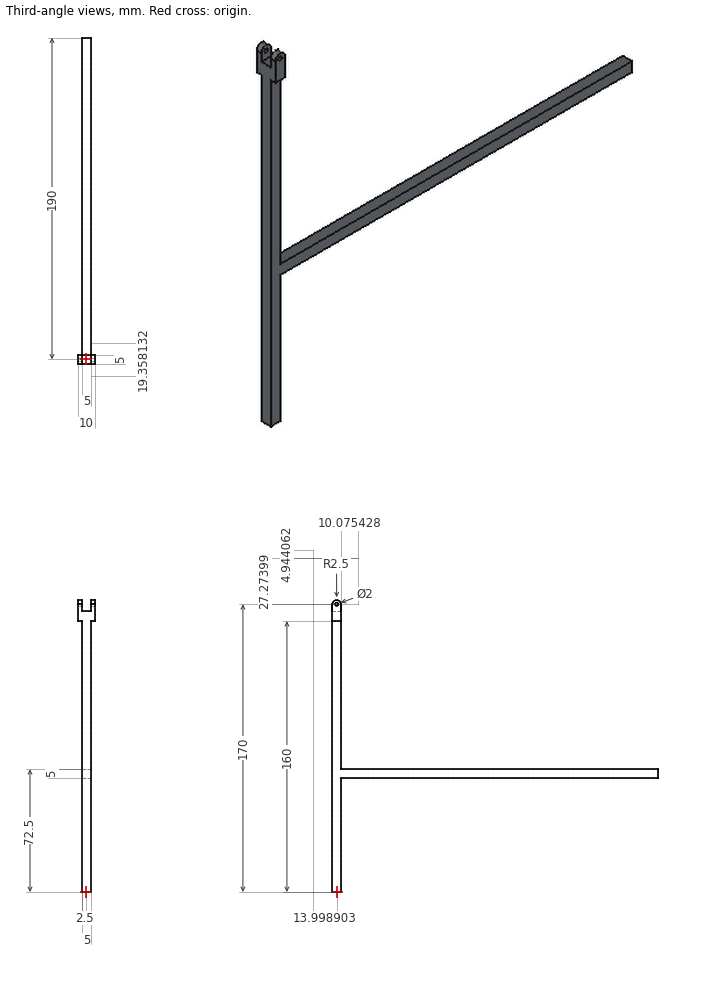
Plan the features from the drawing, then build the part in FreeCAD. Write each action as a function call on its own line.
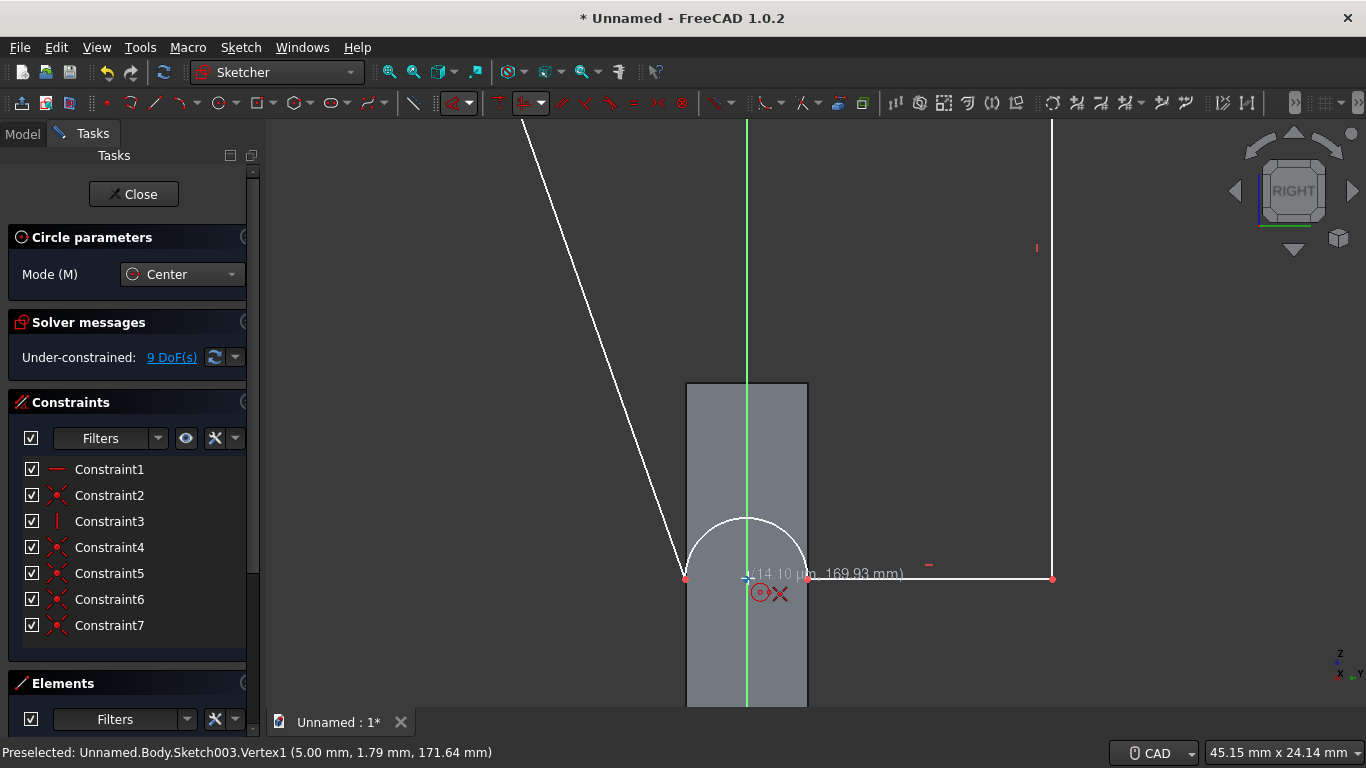
click(747, 578)
click(764, 560)
key(Escape)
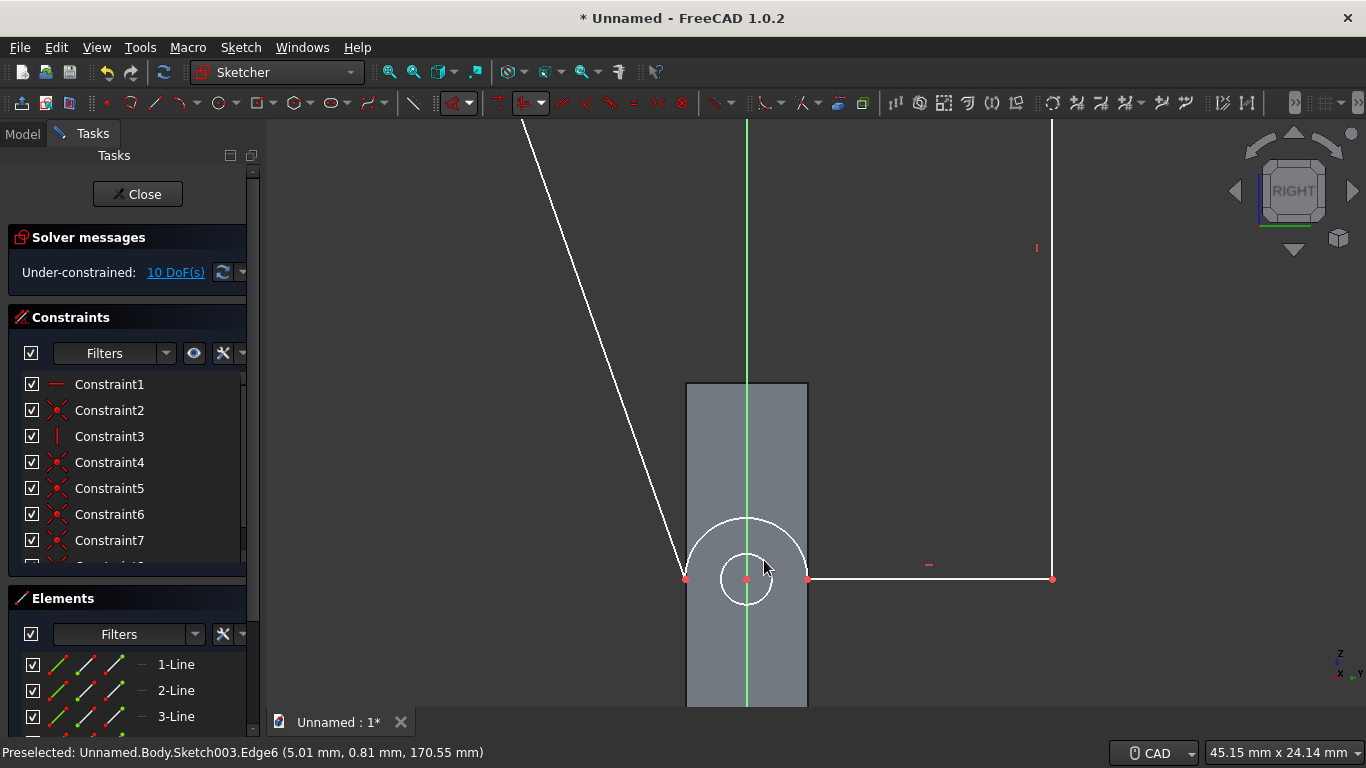
click(746, 579)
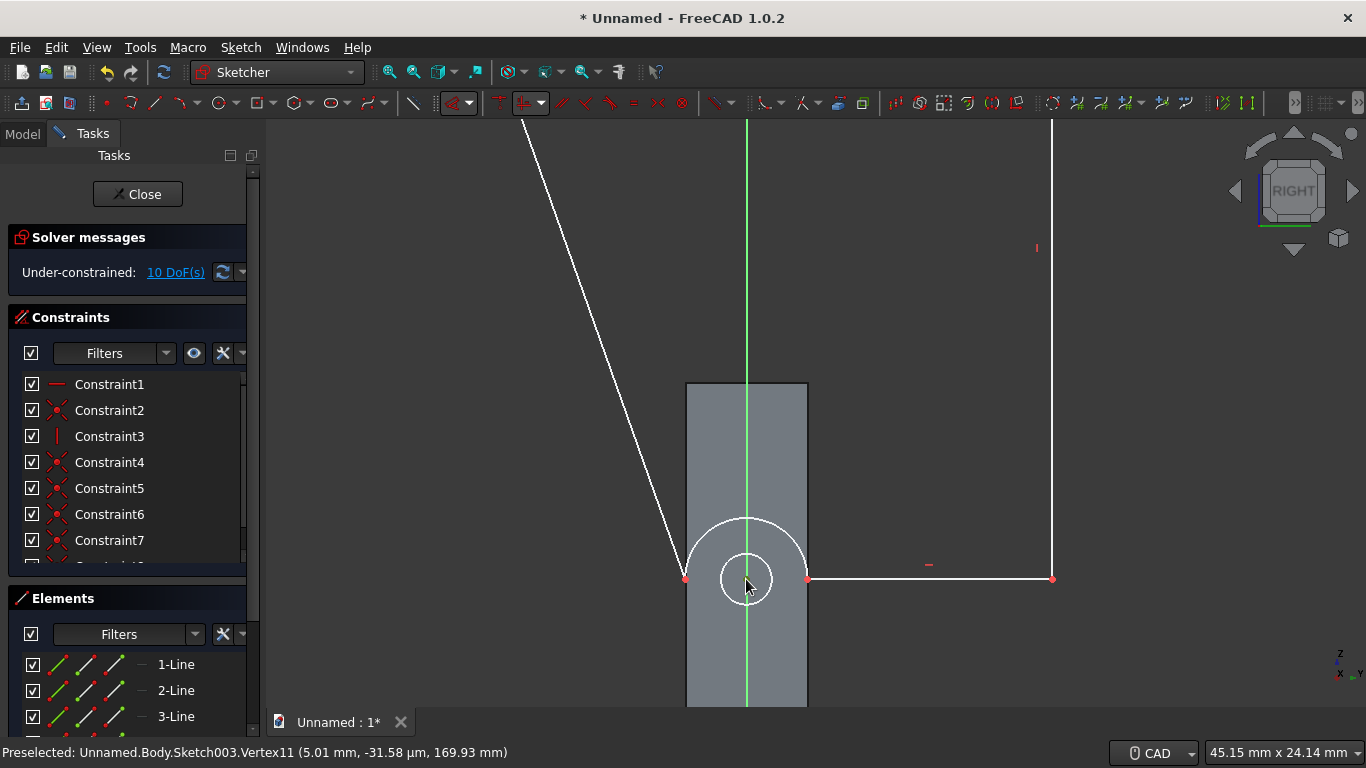
click(747, 641)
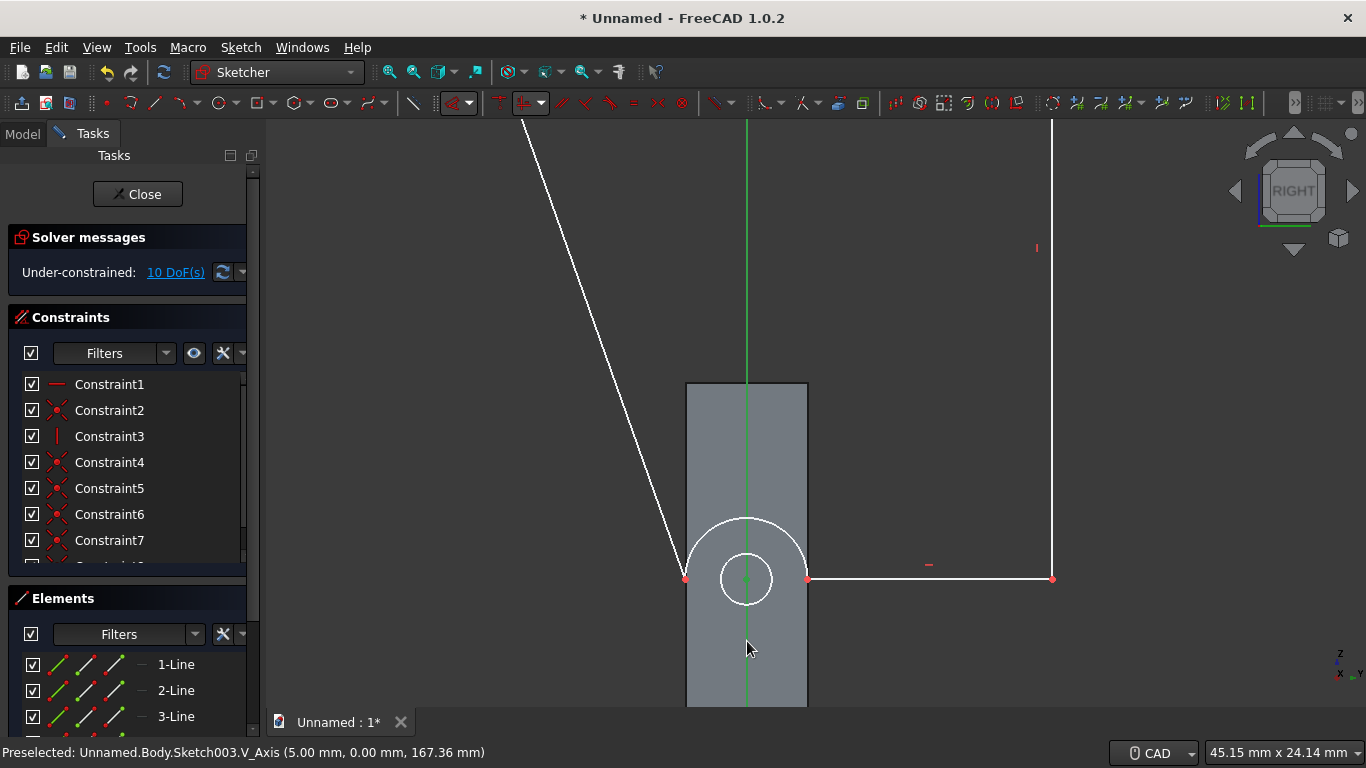
click(500, 104)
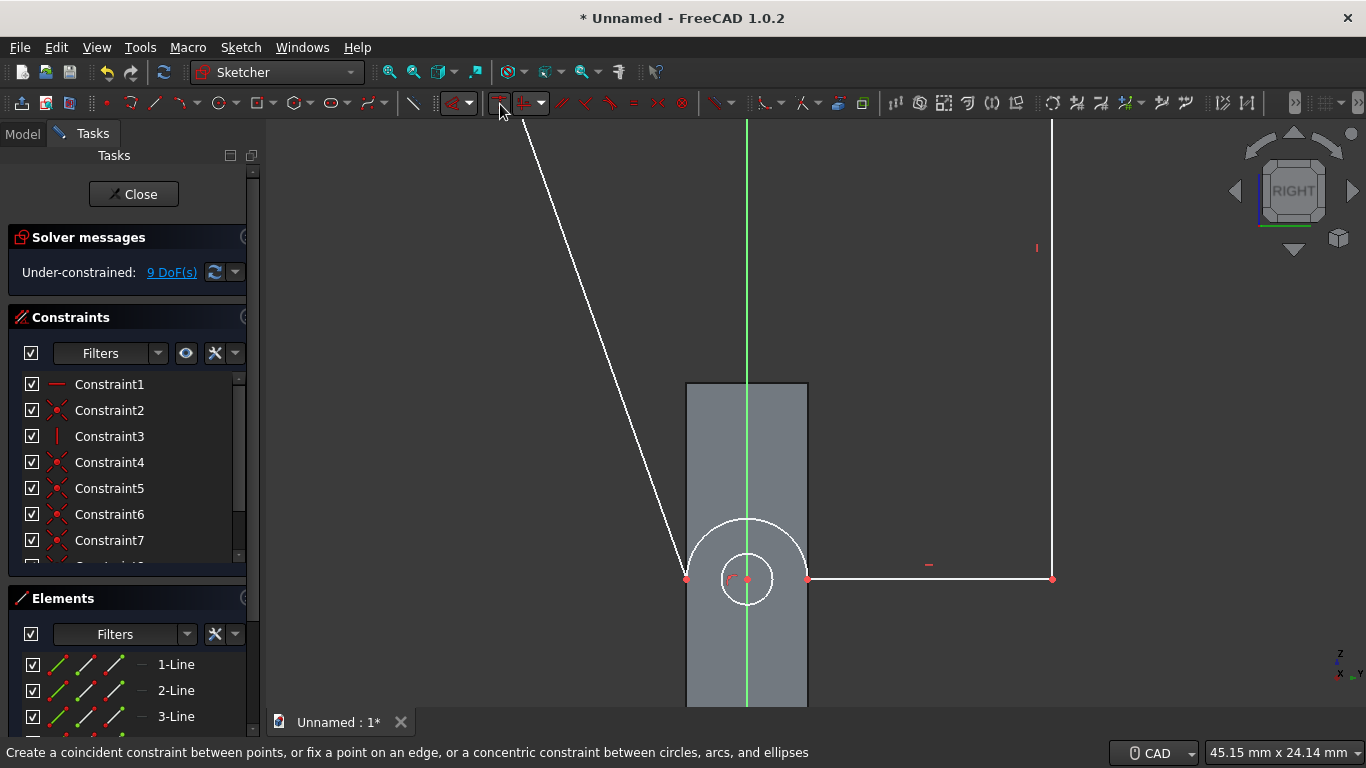
click(783, 530)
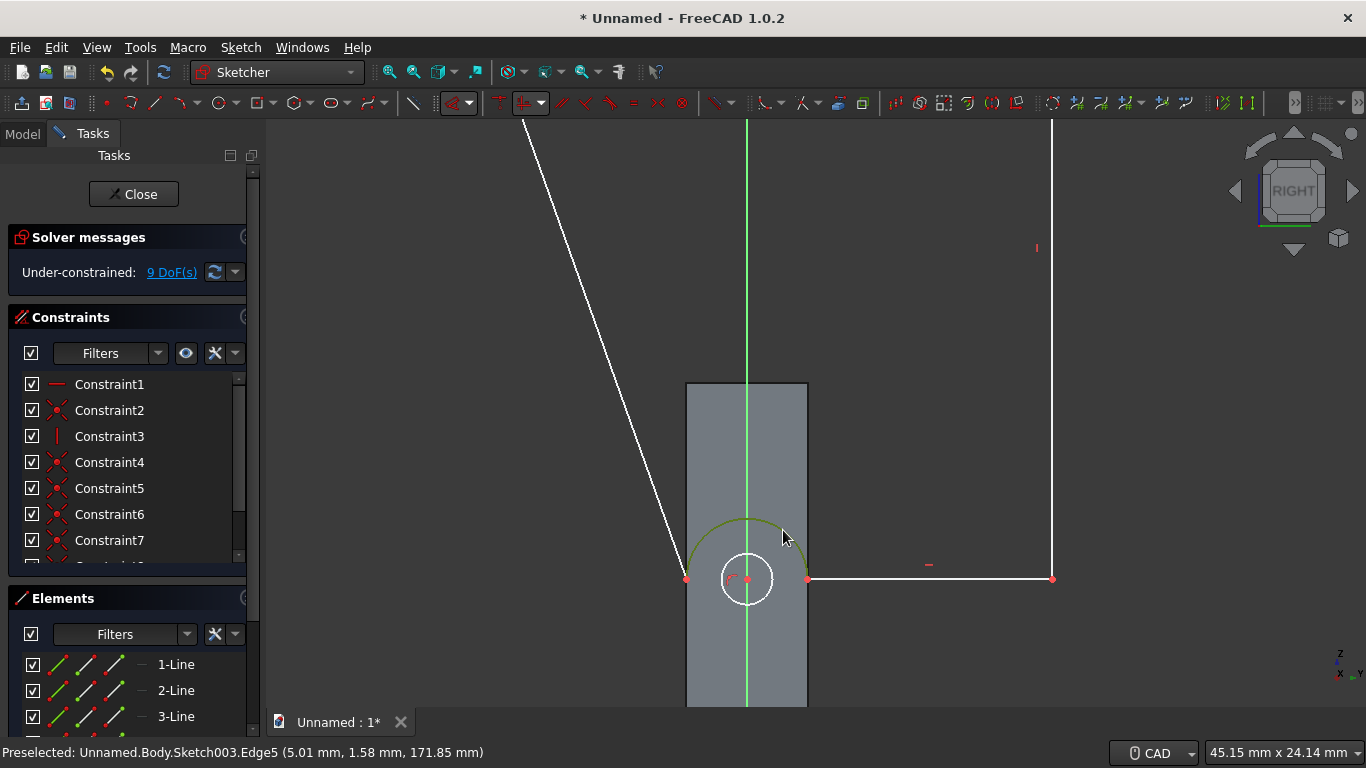
click(472, 104)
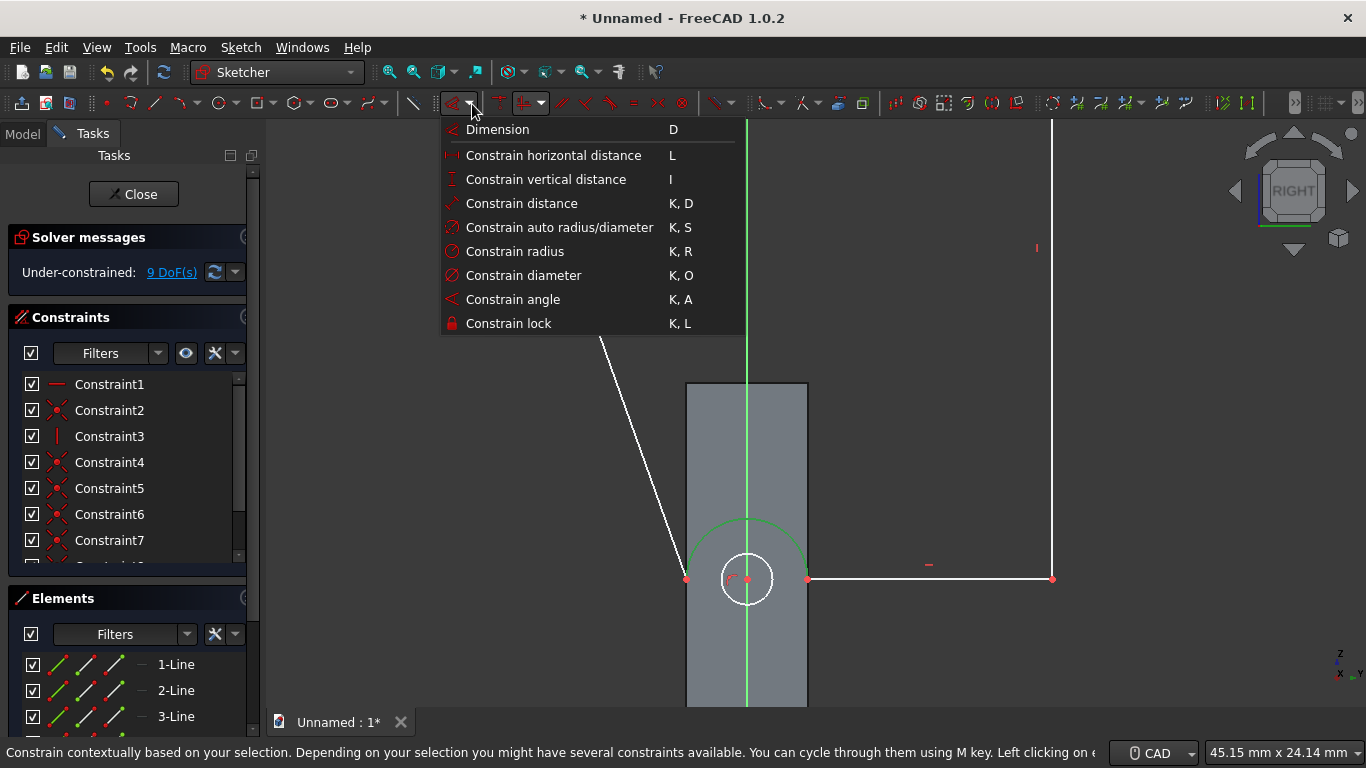
click(593, 251)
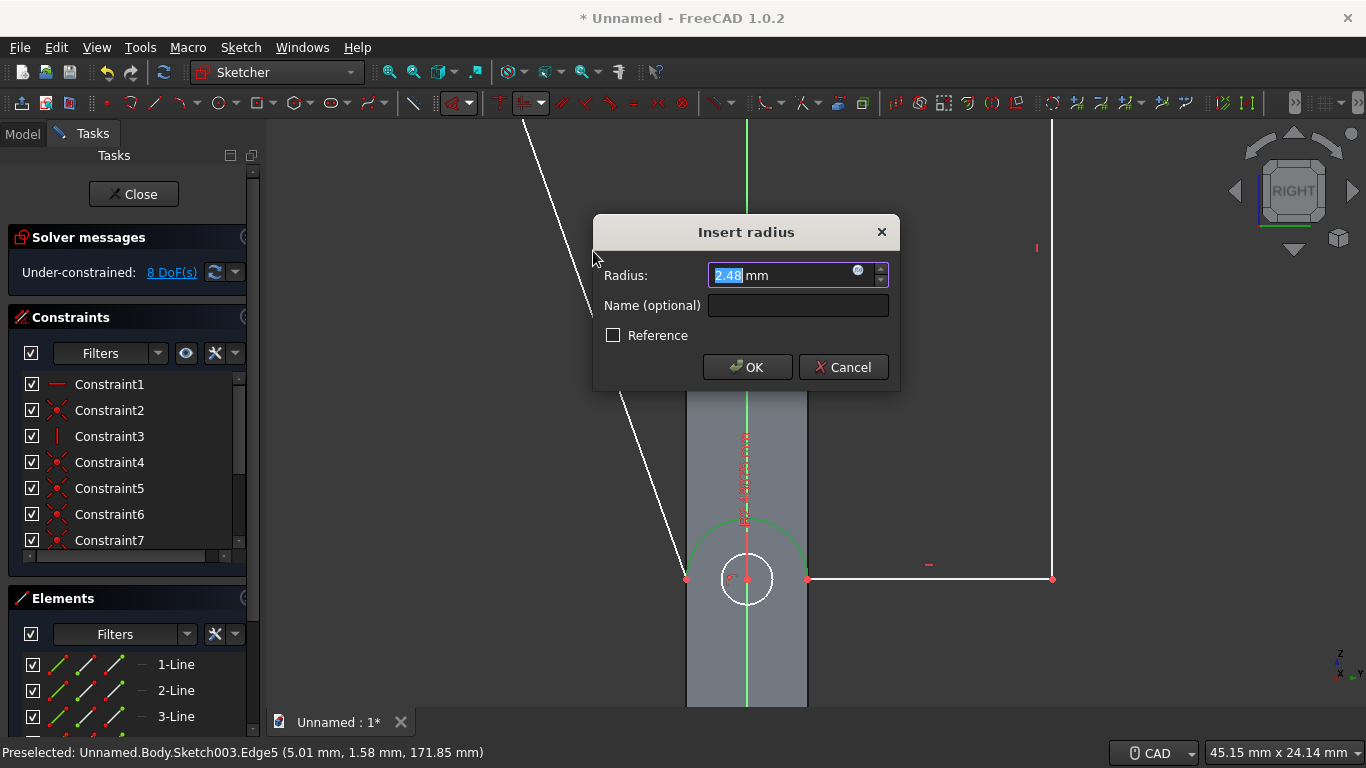
text(2.5)
key(Return)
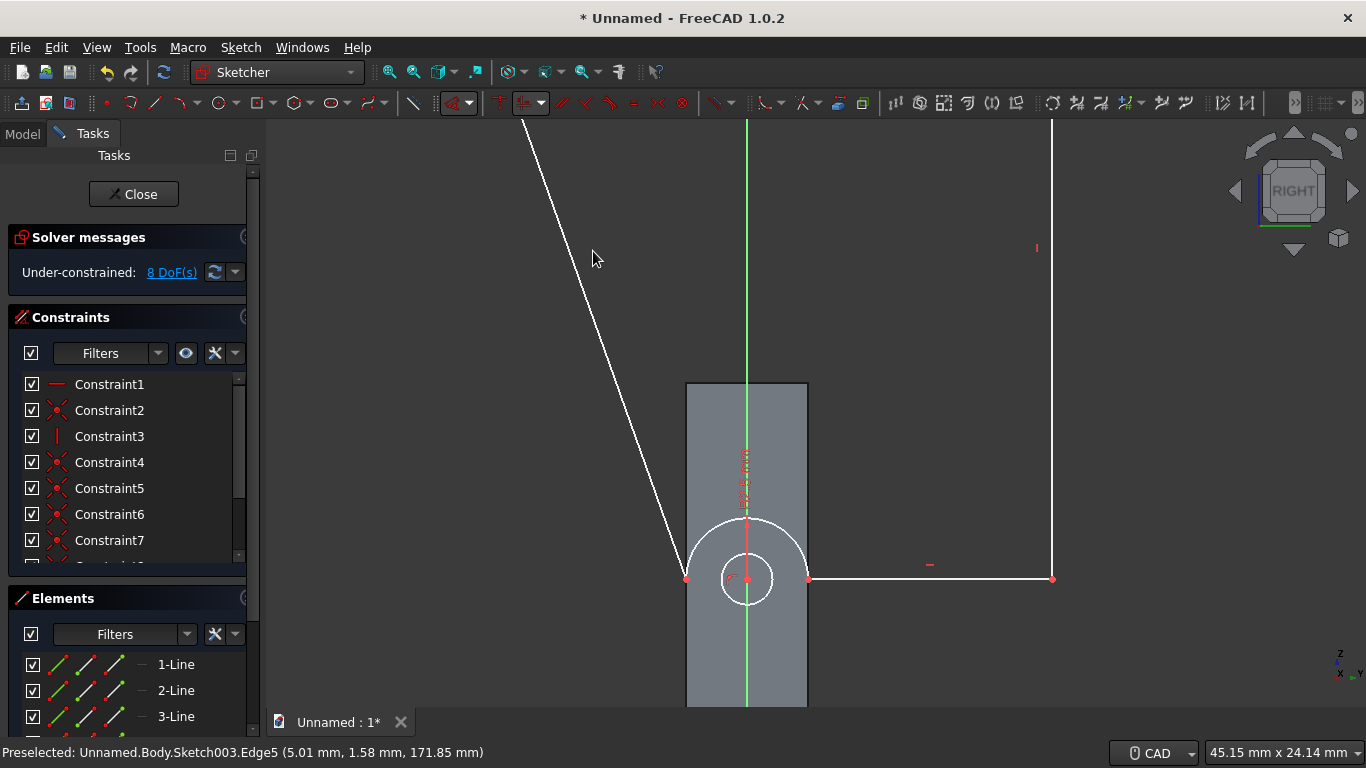
click(765, 561)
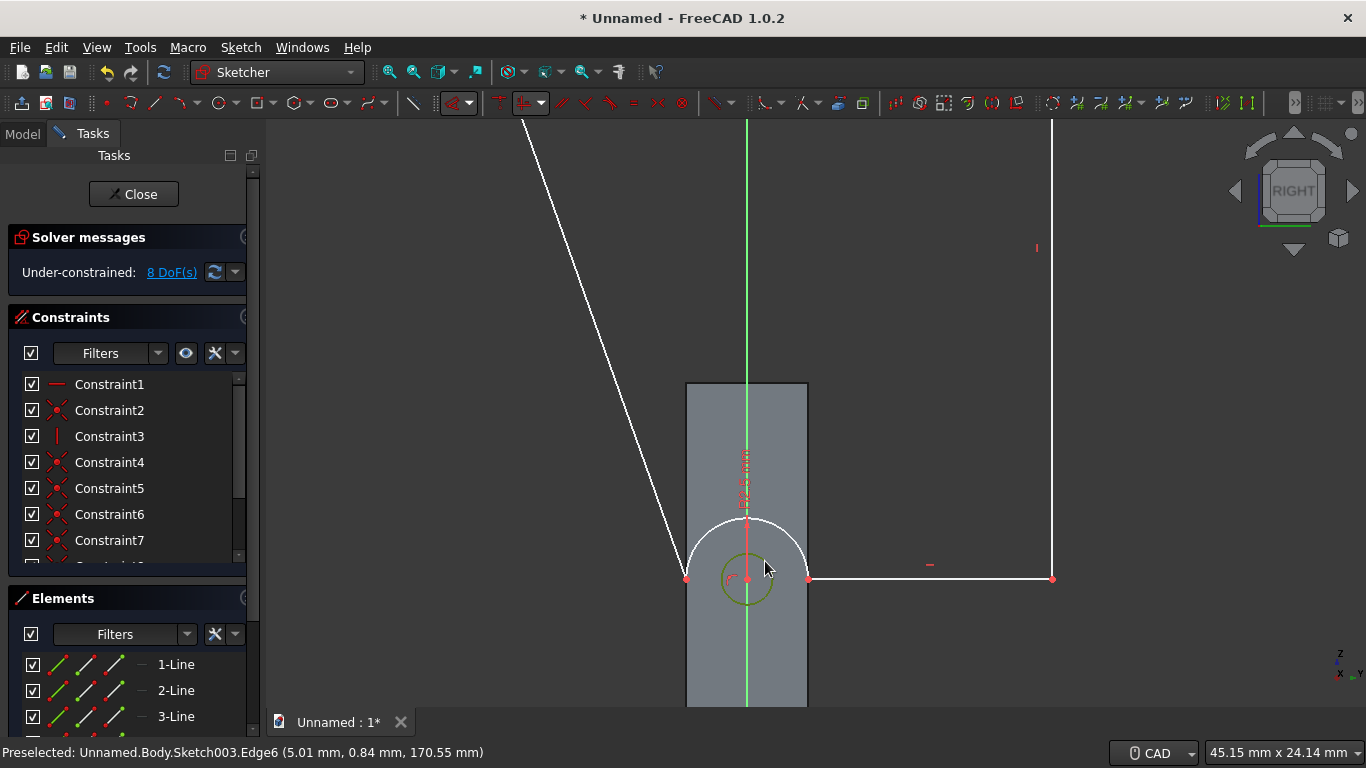
click(472, 104)